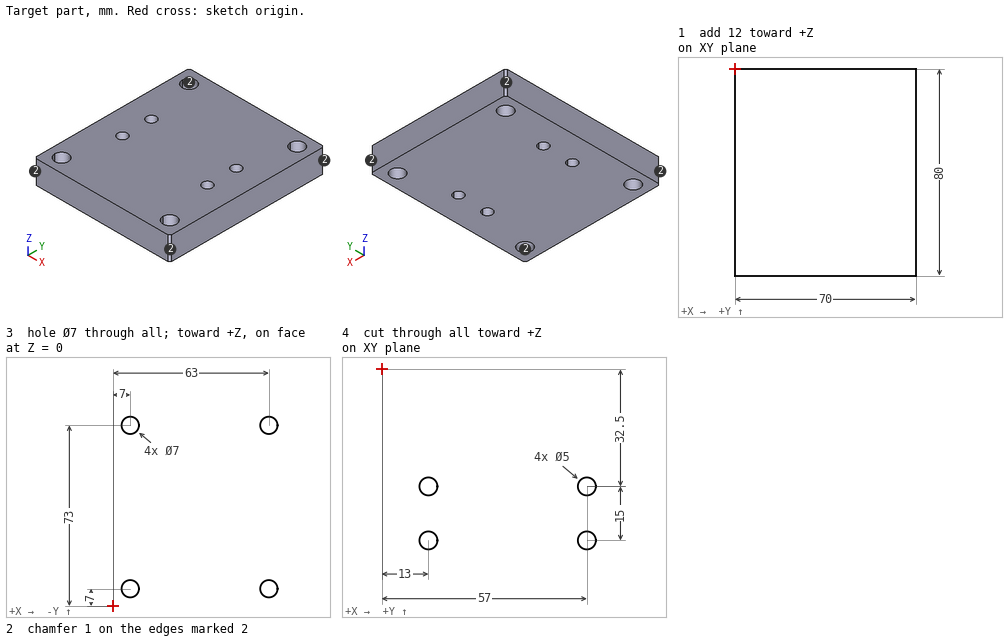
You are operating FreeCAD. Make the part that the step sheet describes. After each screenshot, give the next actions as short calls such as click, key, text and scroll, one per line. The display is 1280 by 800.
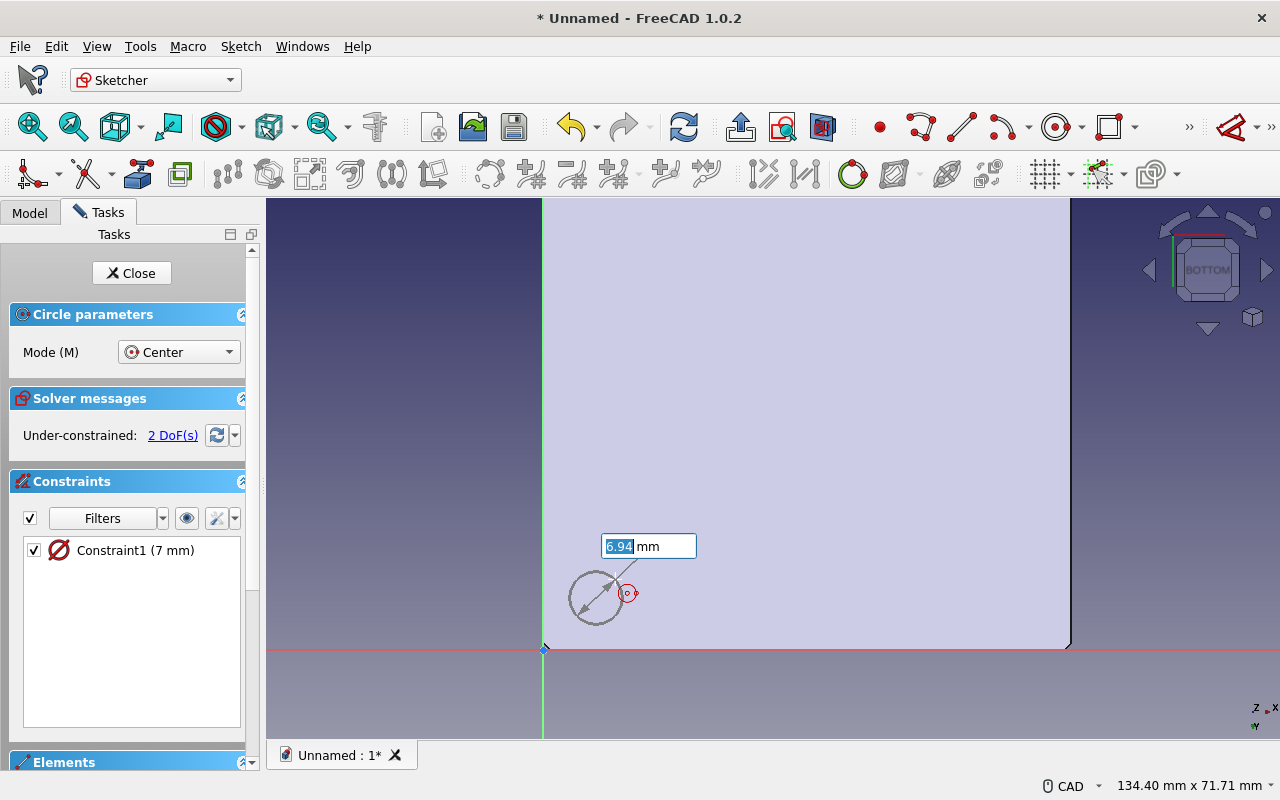
text(7)
key(Return)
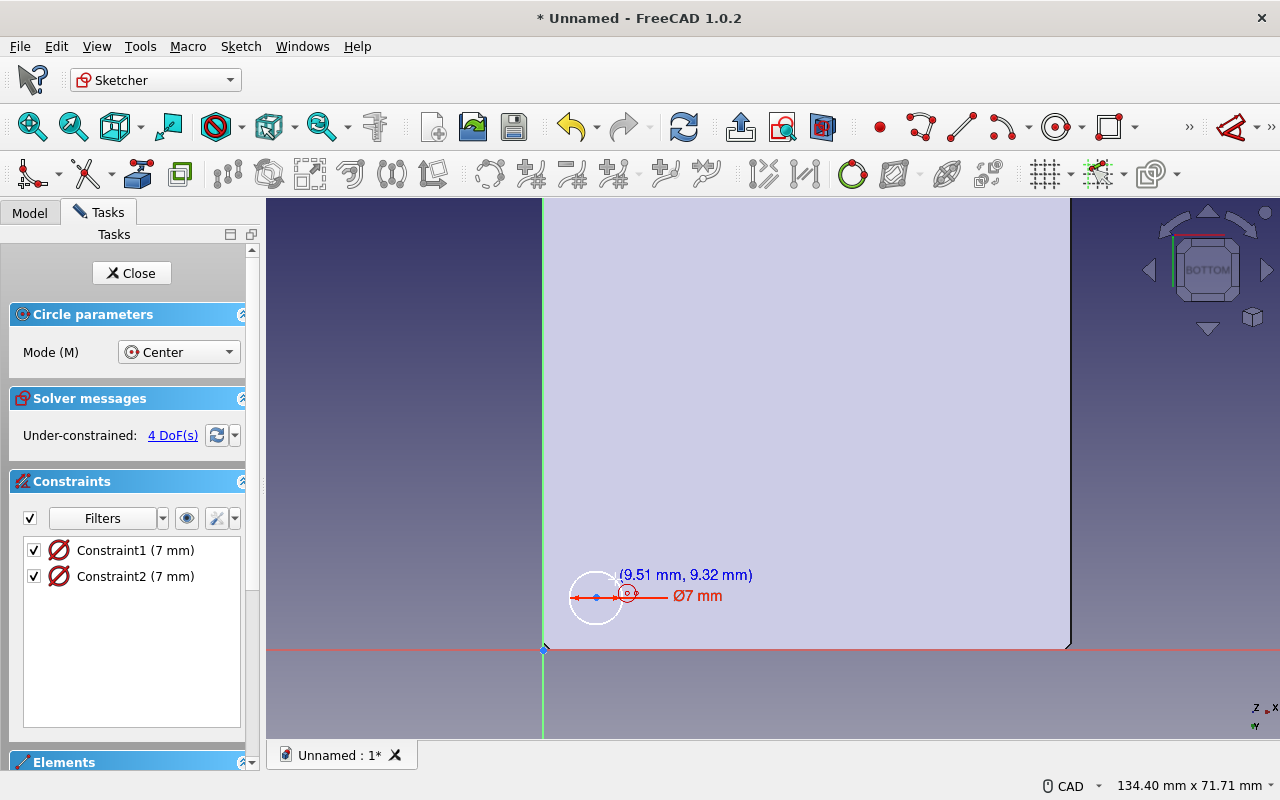
scroll(596, 598, down, 3)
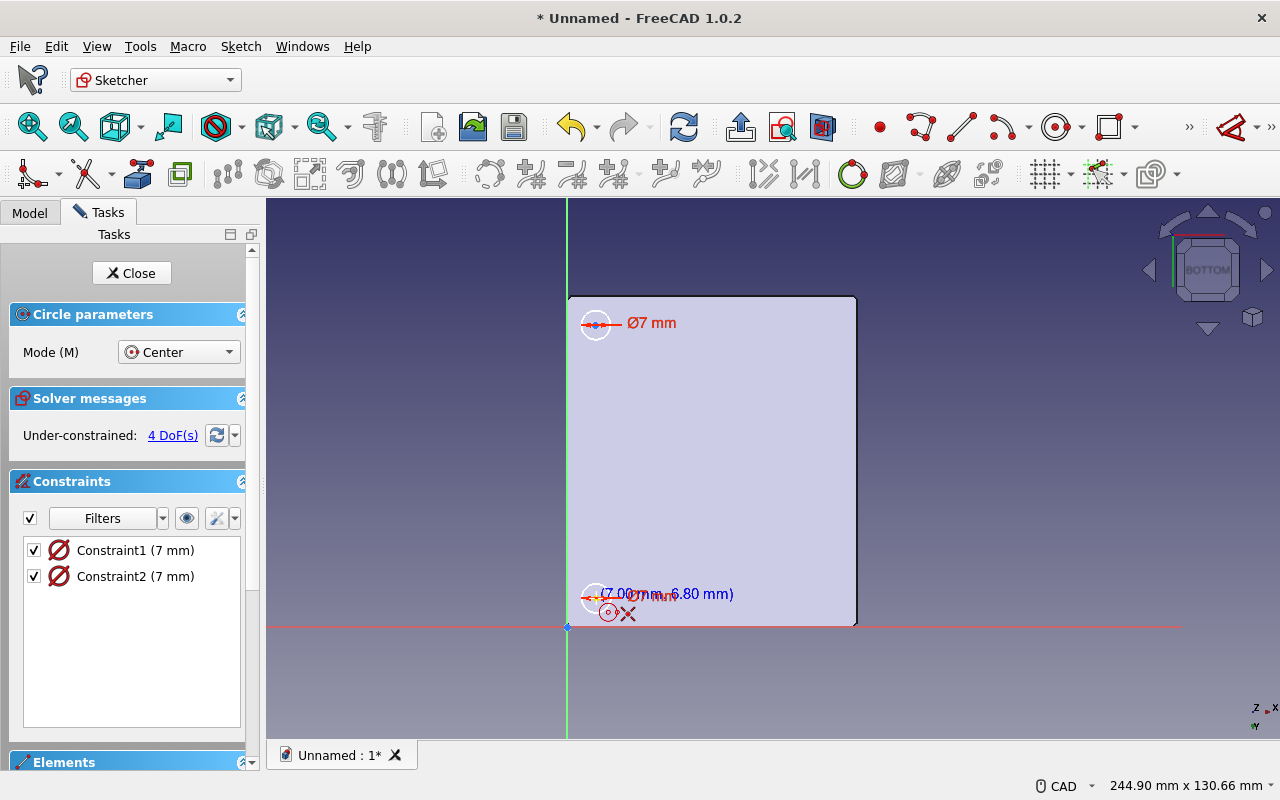
scroll(828, 325, up, 3)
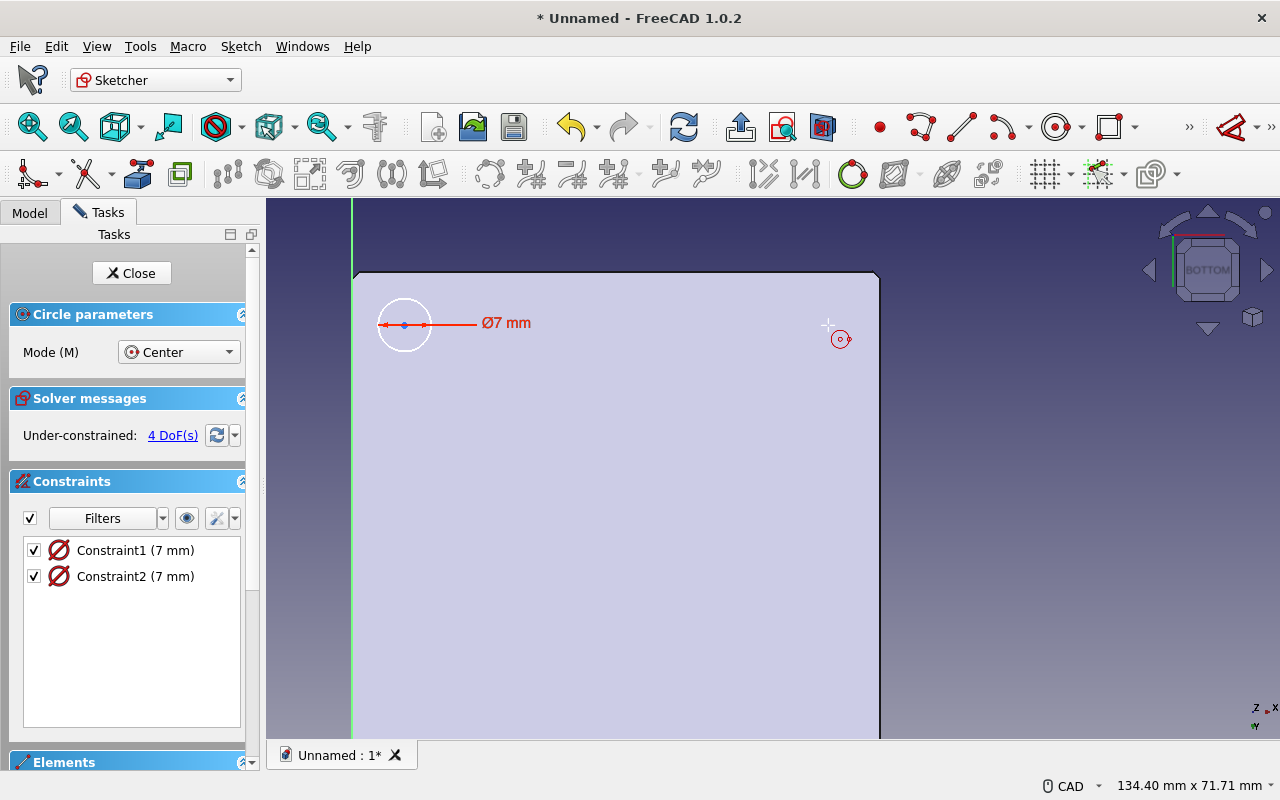
click(828, 324)
move(846, 306)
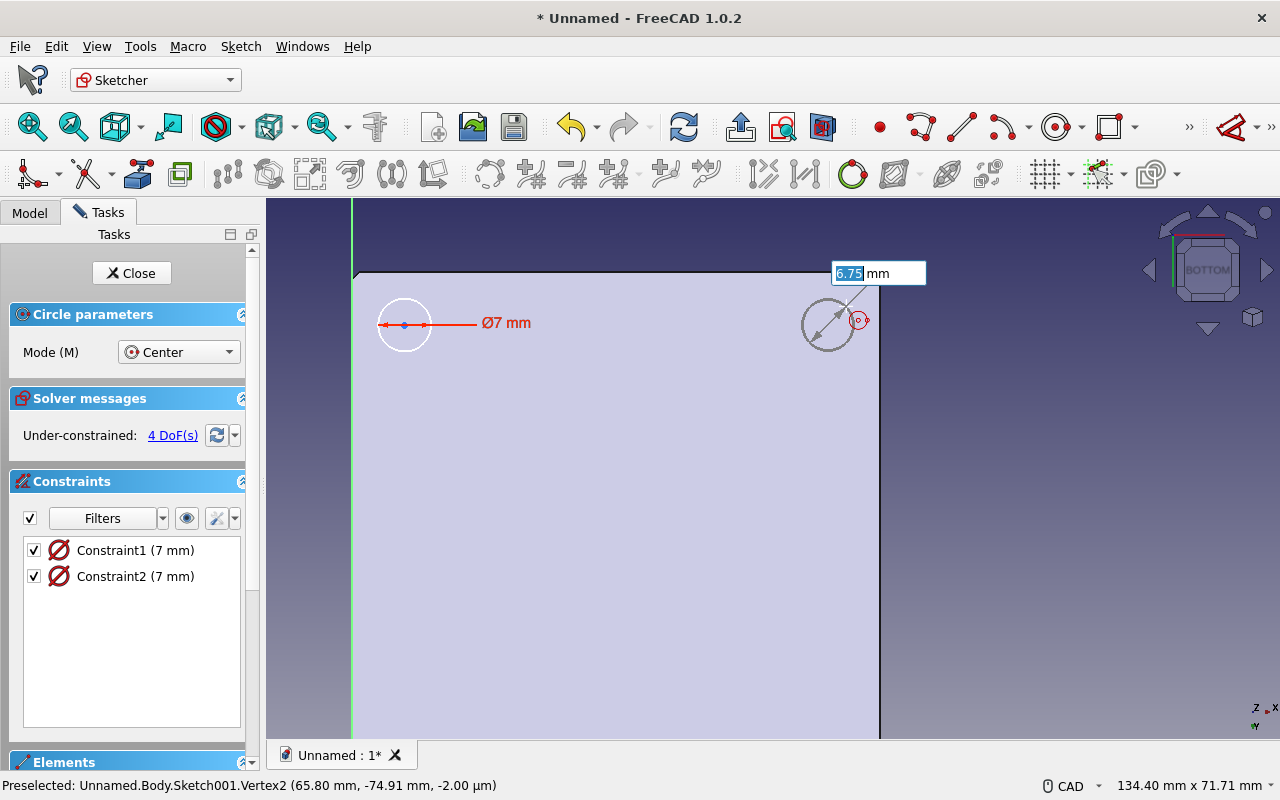
text(7)
key(Return)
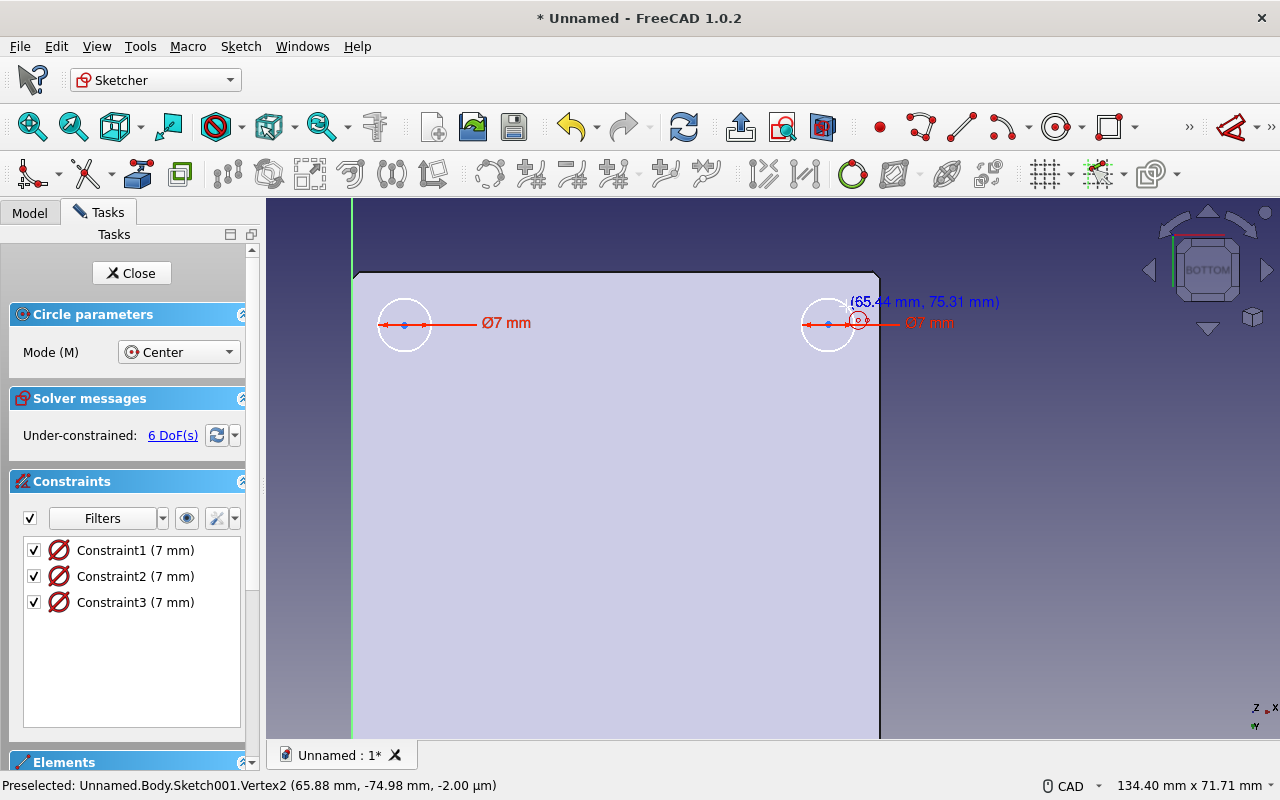
scroll(828, 325, down, 3)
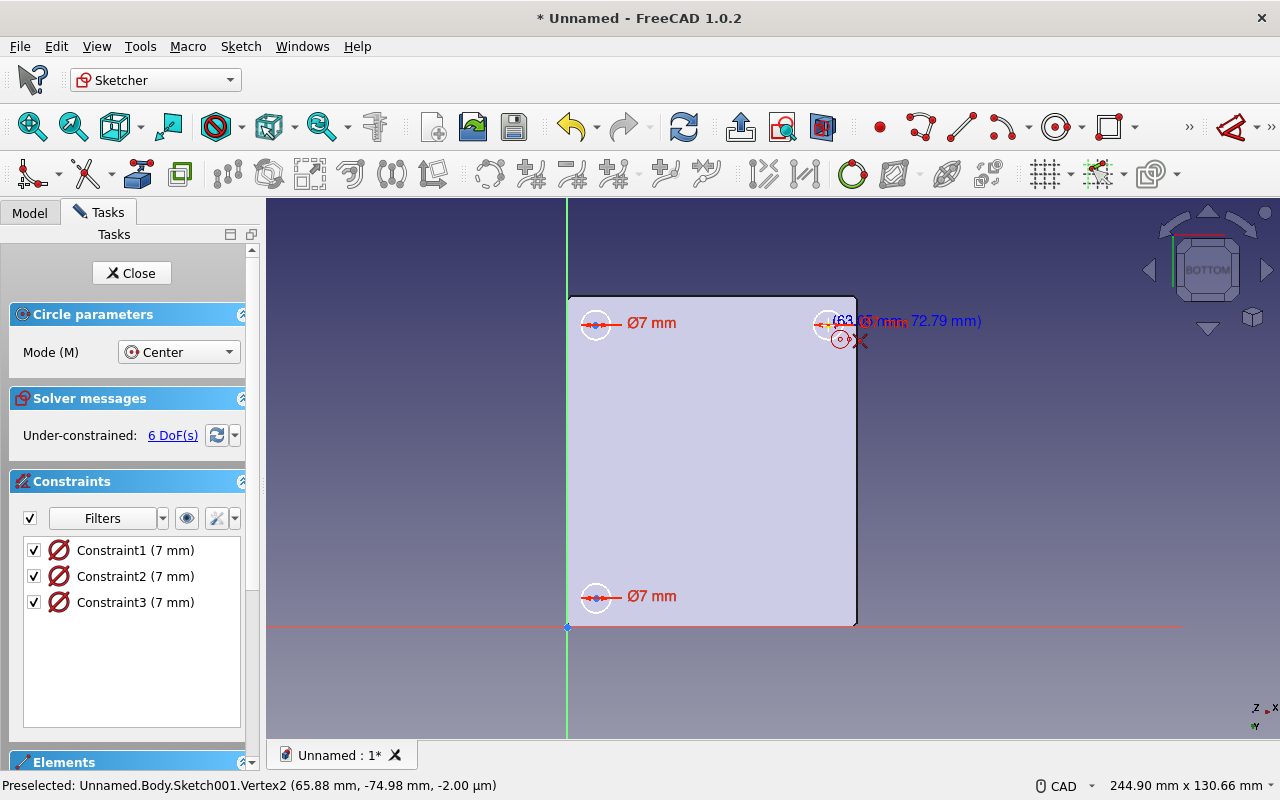
scroll(828, 598, up, 3)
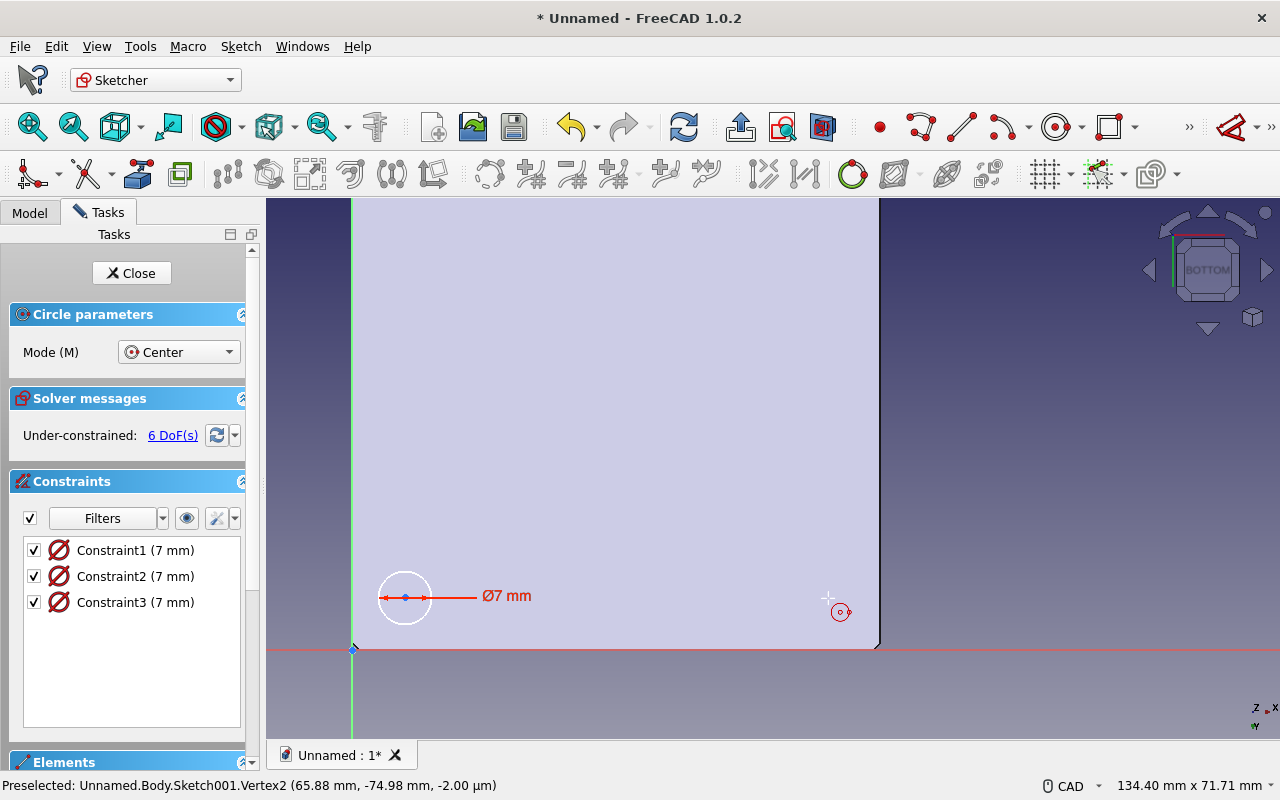
click(828, 597)
move(846, 579)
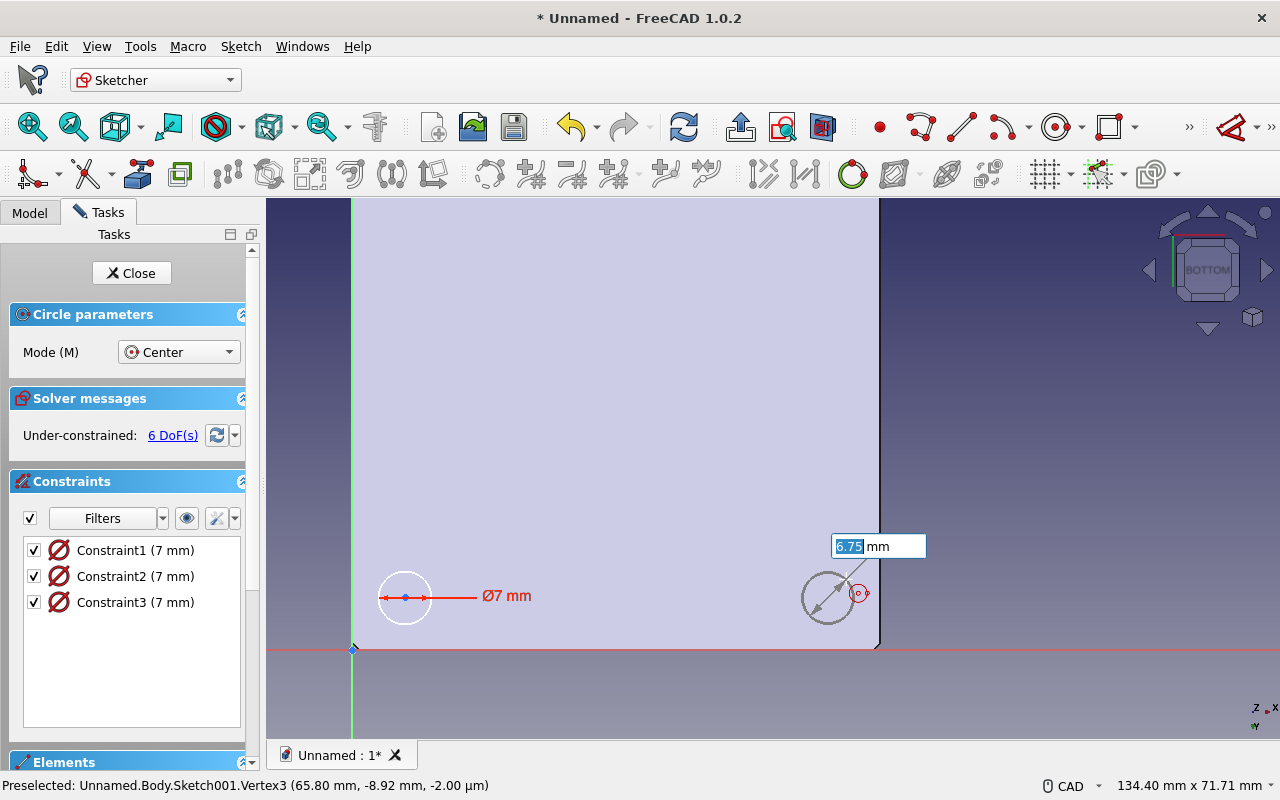
text(7)
key(Return)
key(Escape)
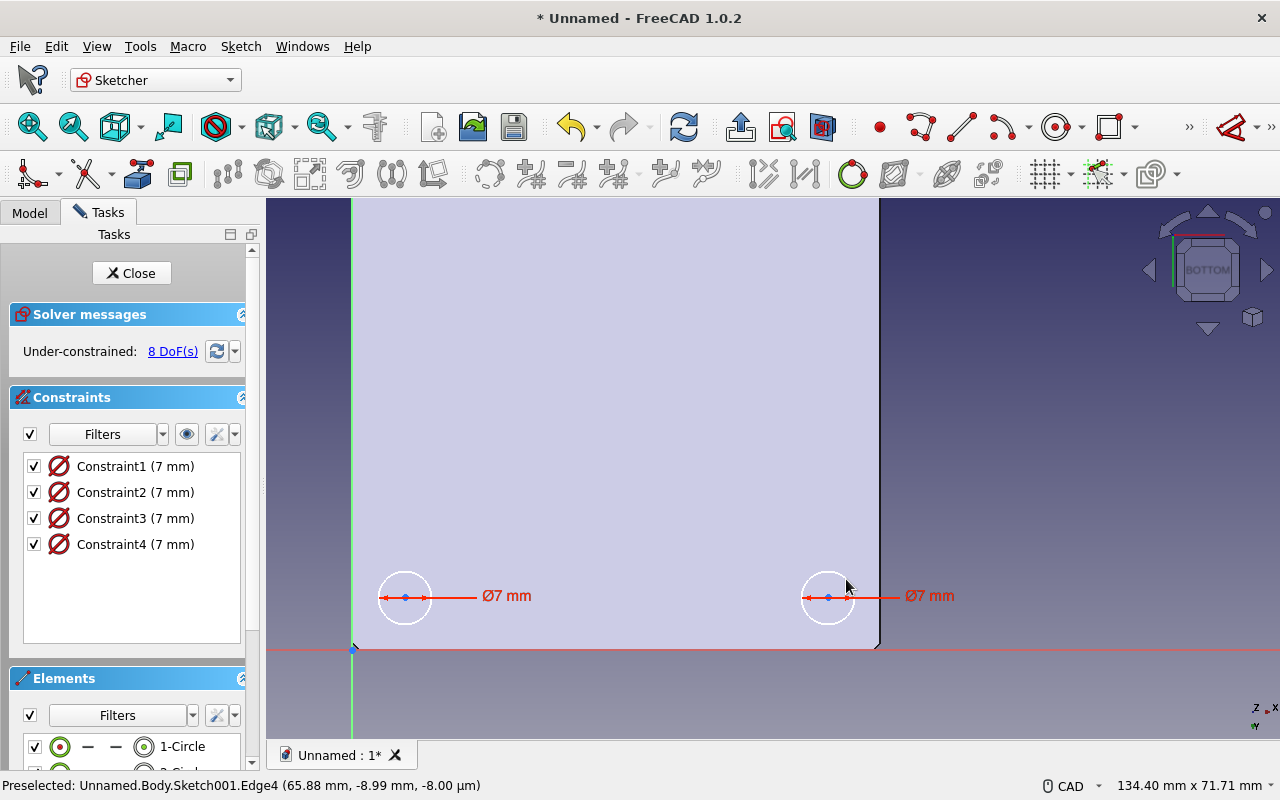
scroll(828, 598, down, 3)